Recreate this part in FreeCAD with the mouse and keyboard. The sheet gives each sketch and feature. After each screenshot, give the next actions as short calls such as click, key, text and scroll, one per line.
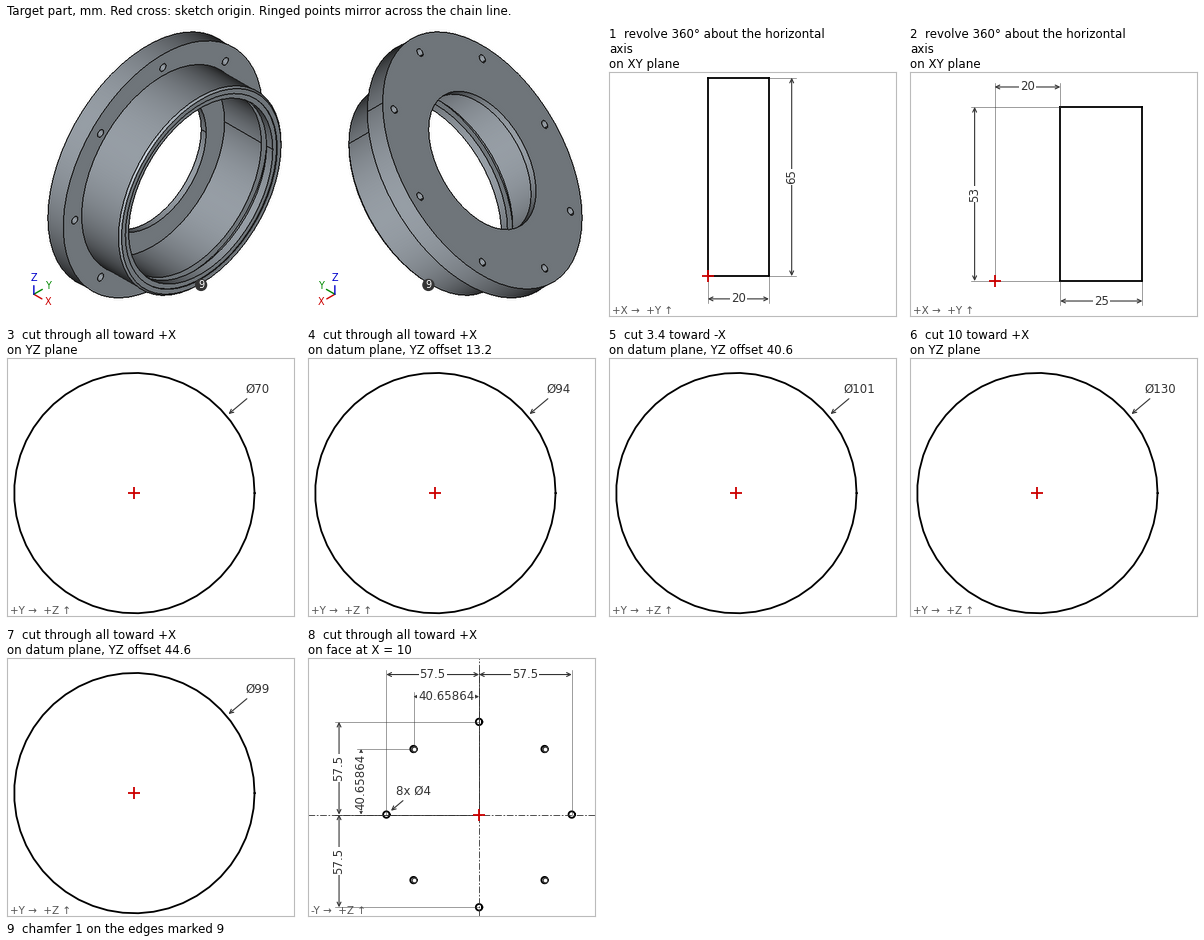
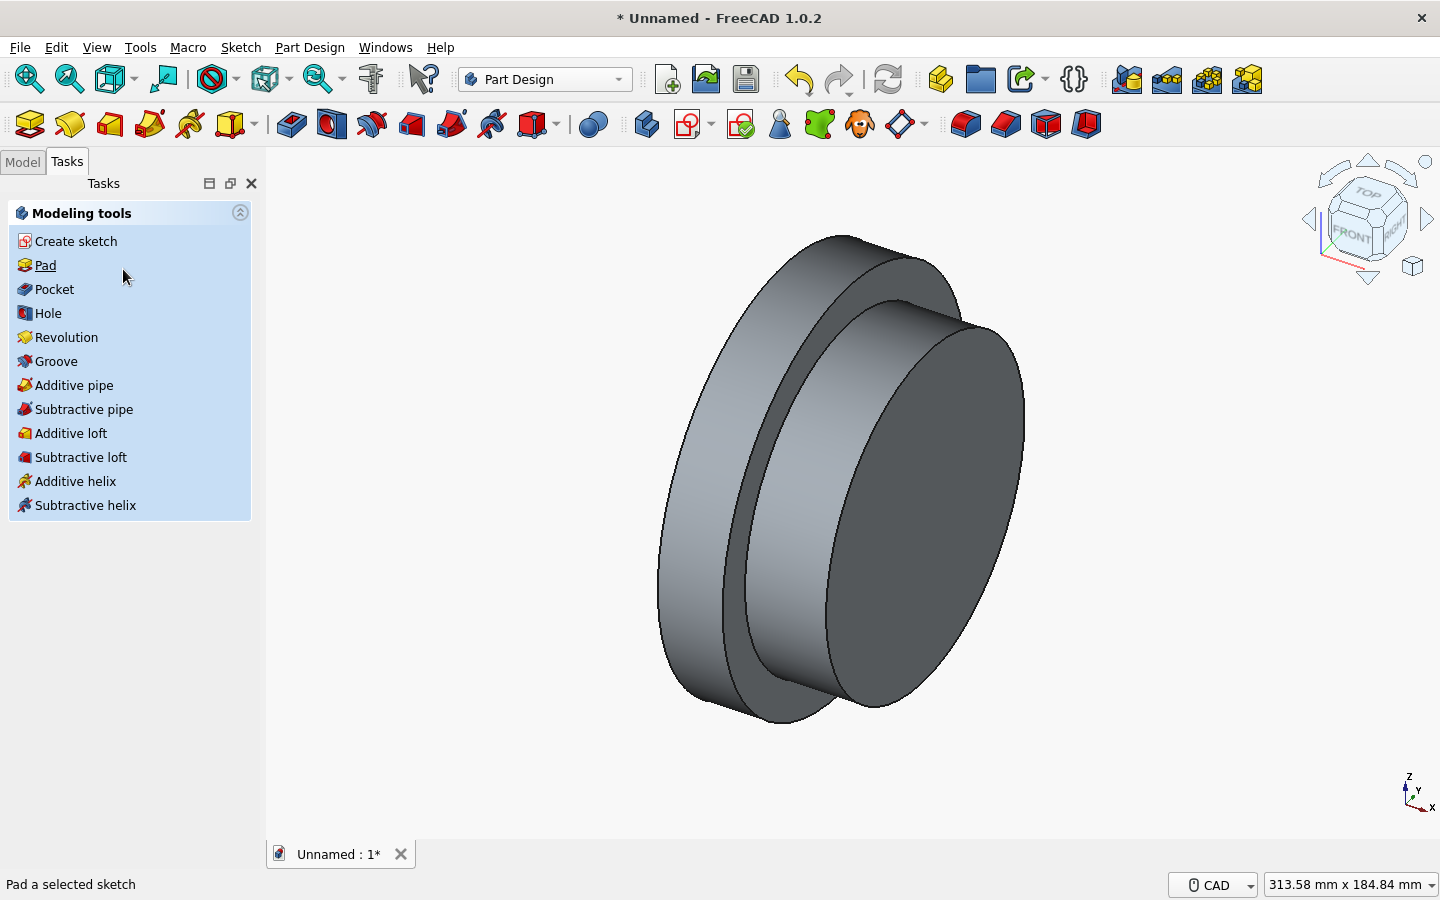
click(292, 124)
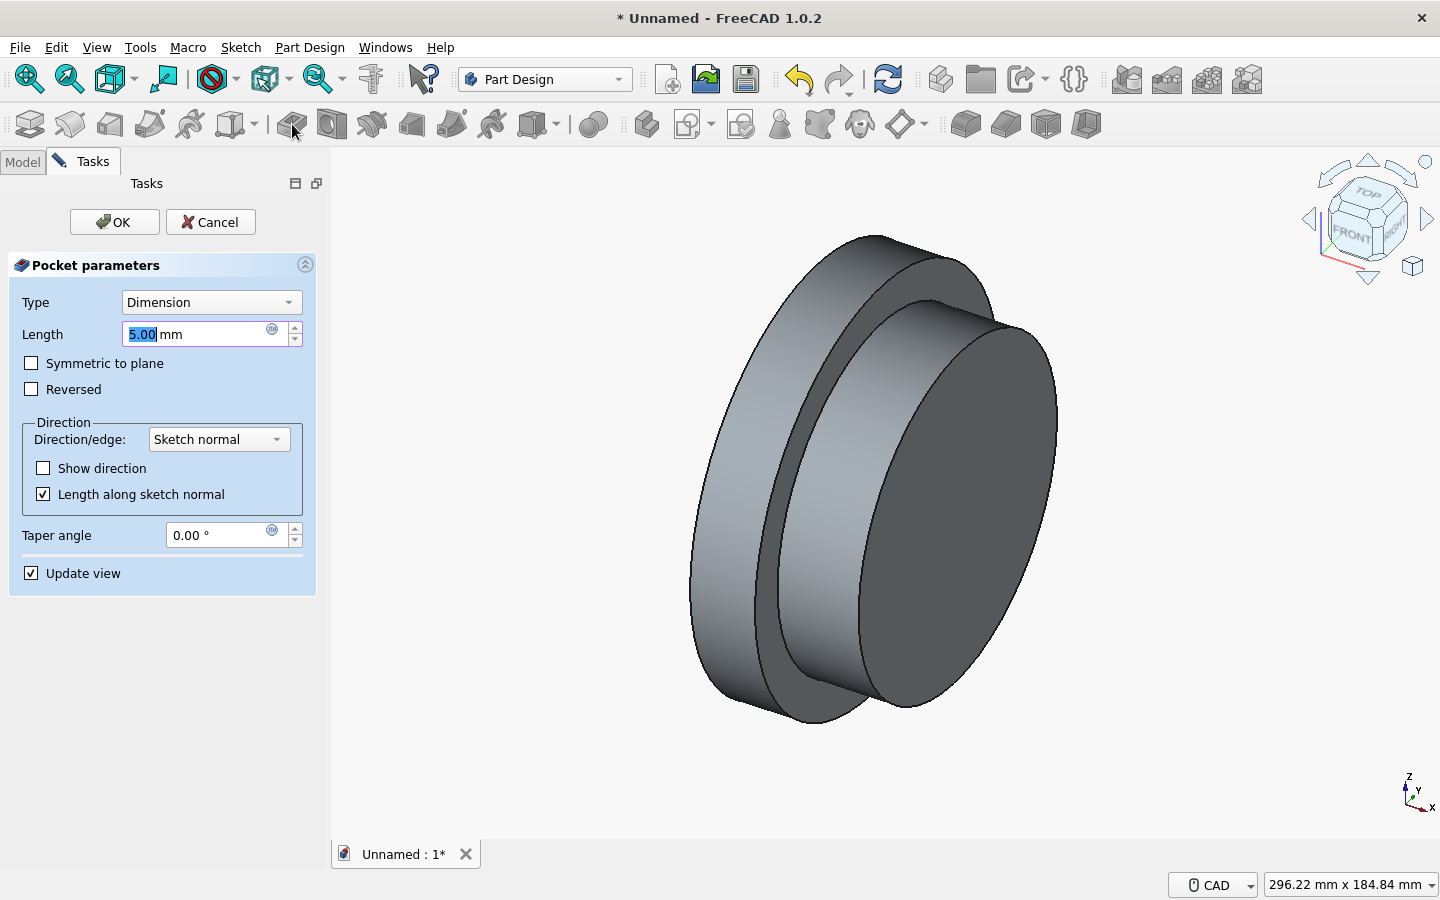
click(212, 302)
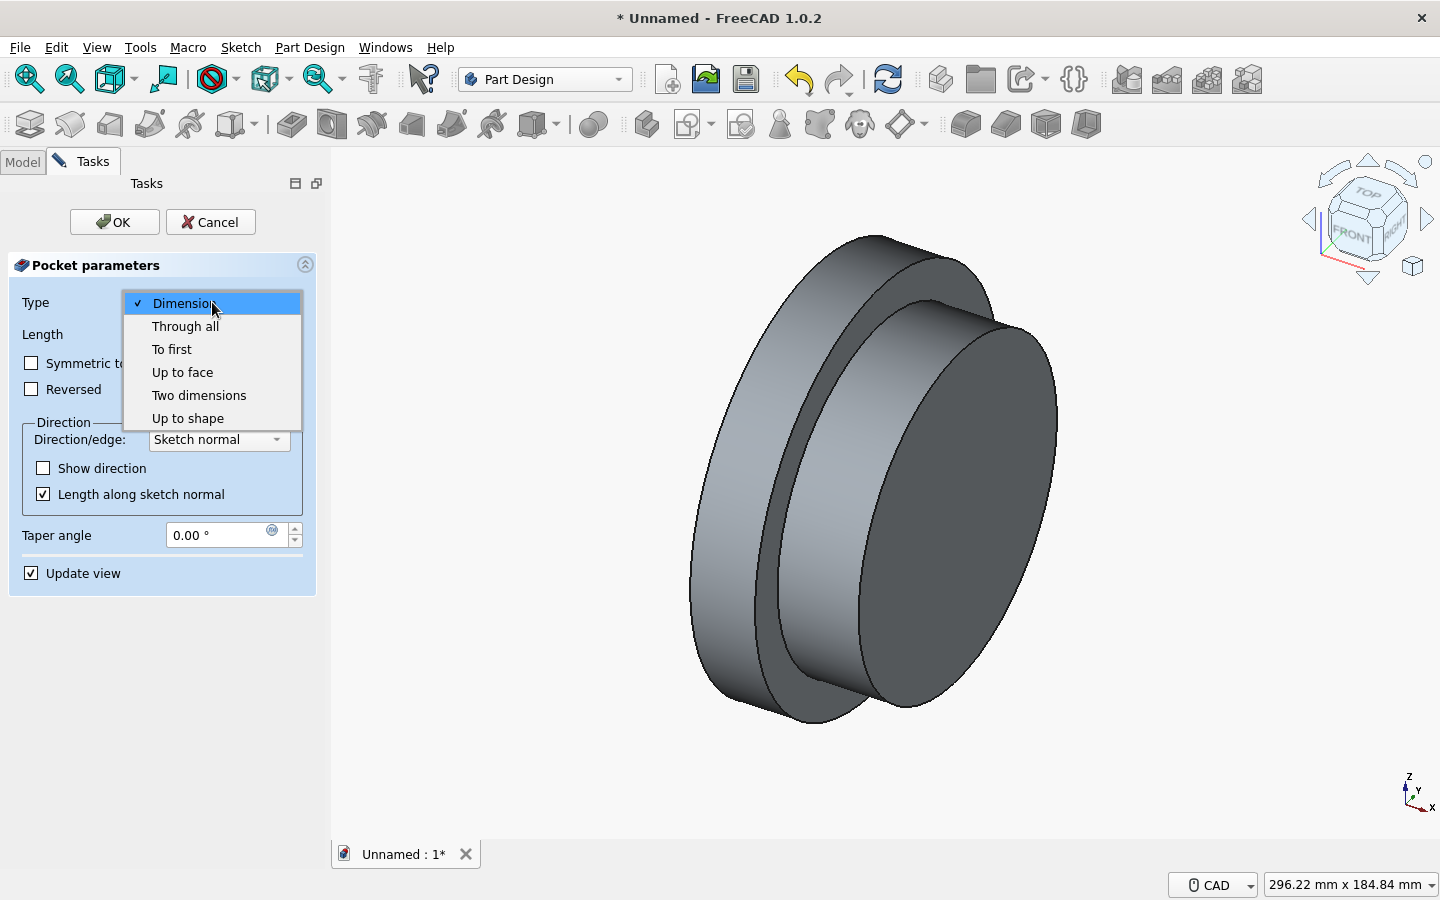
click(212, 326)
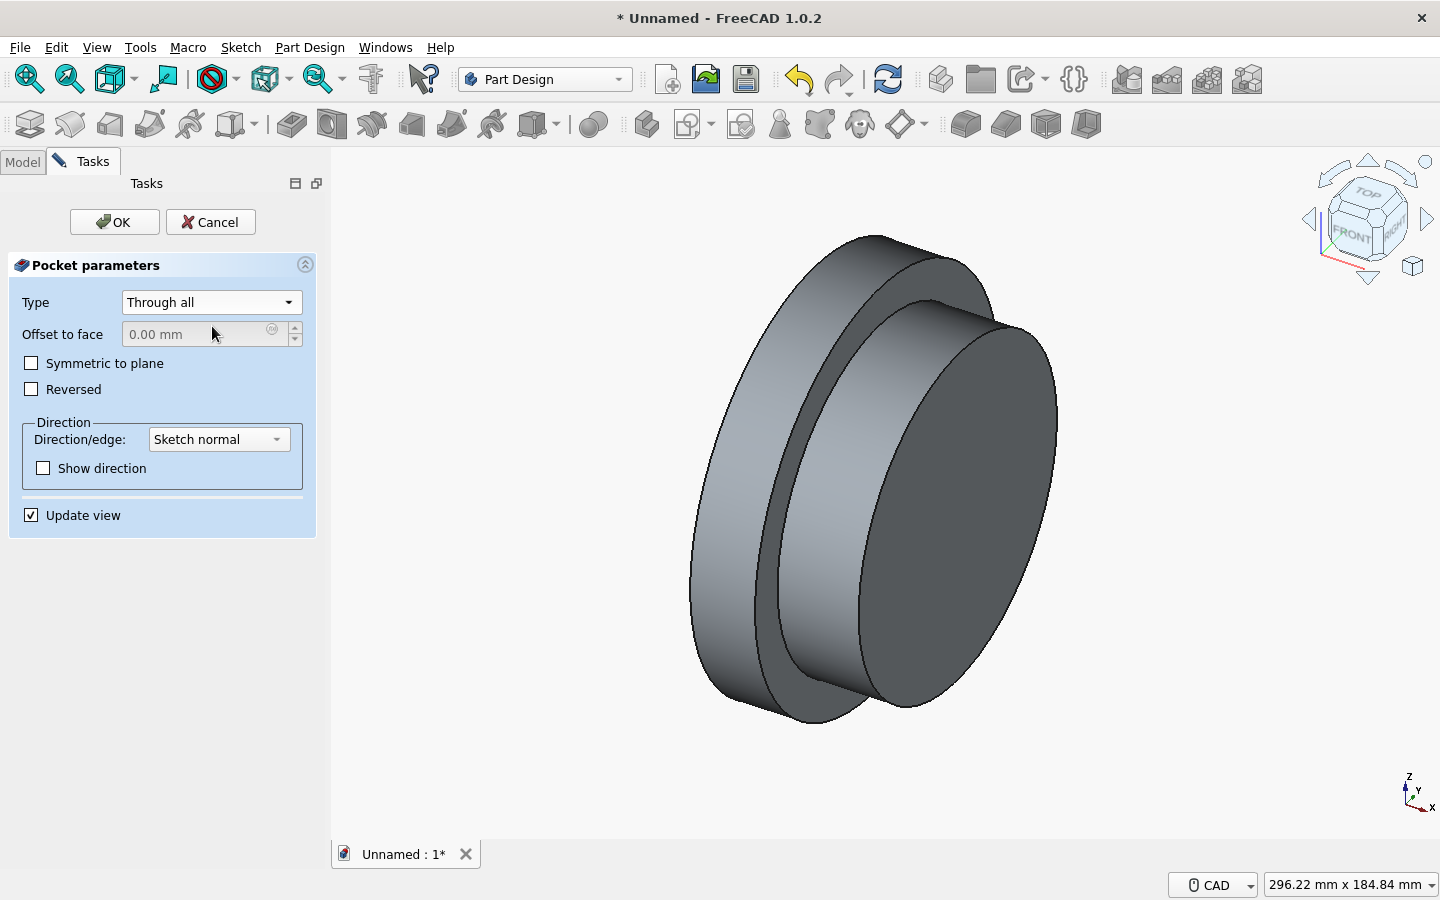
click(30, 389)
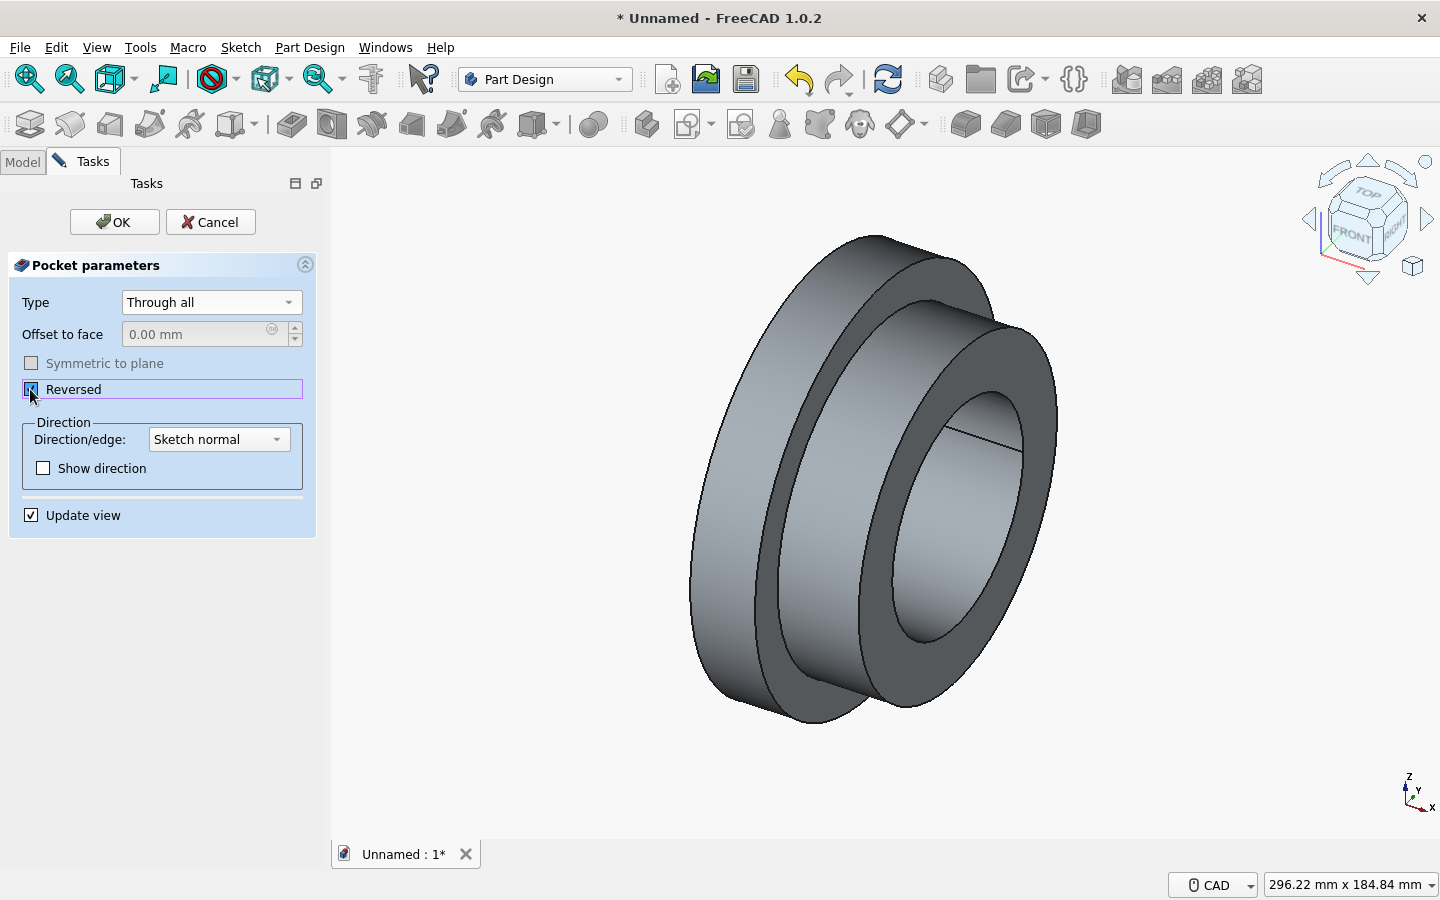
click(115, 222)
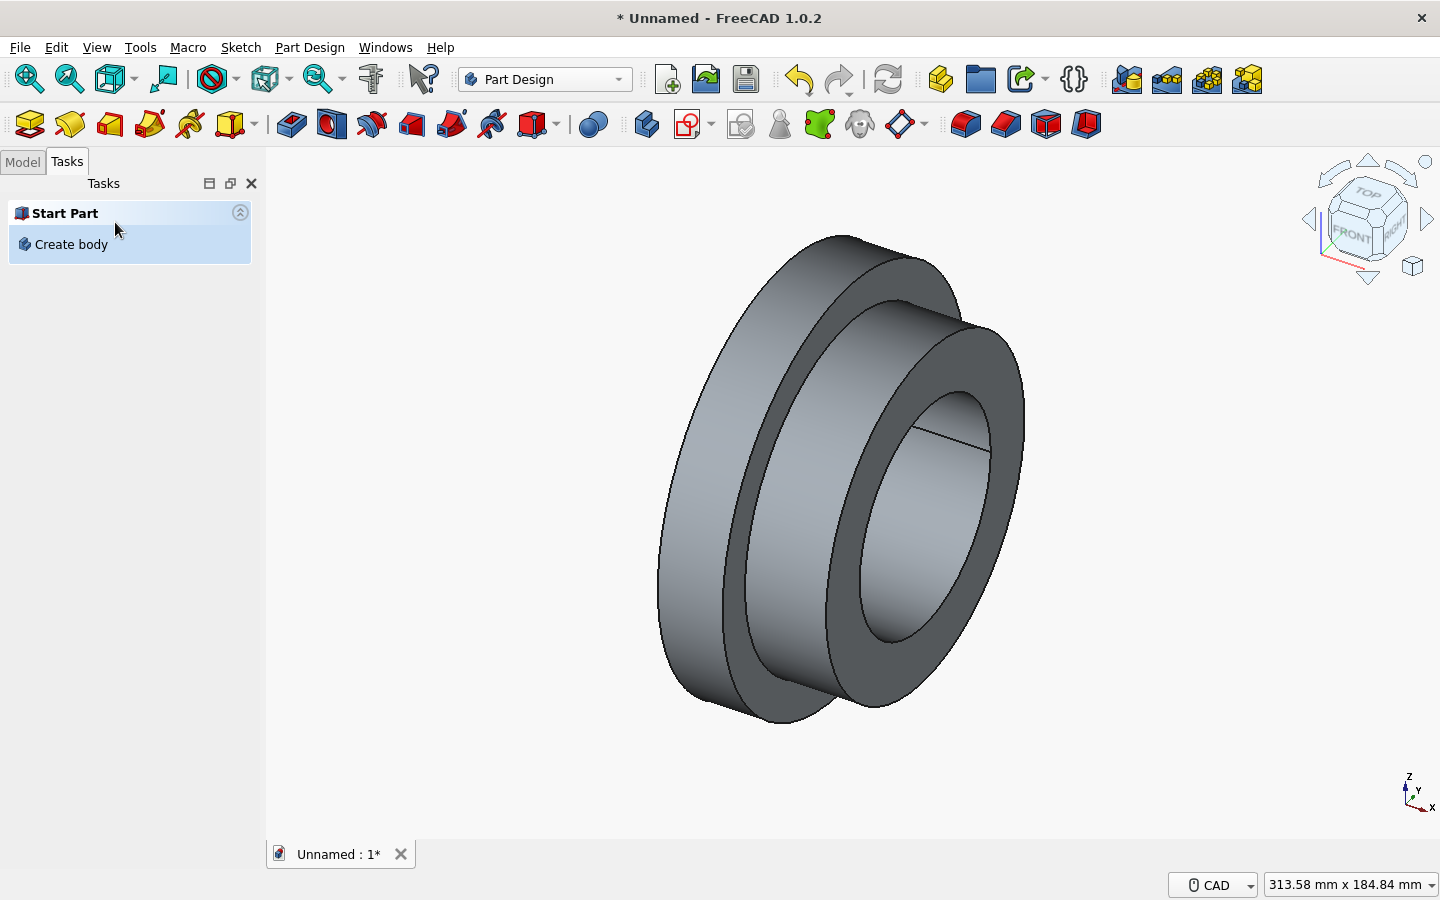
click(23, 161)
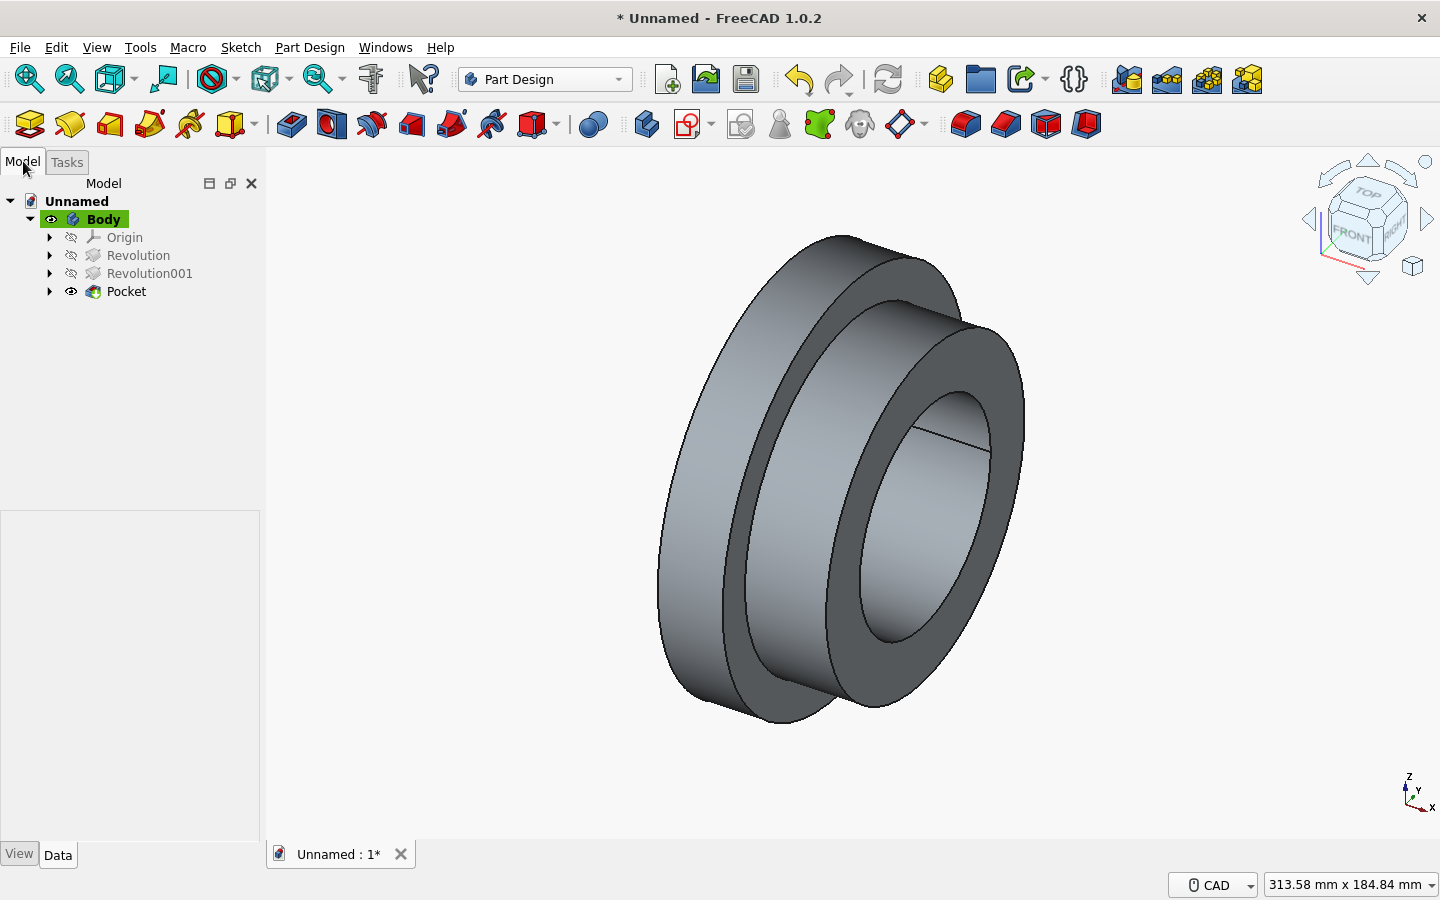
click(50, 237)